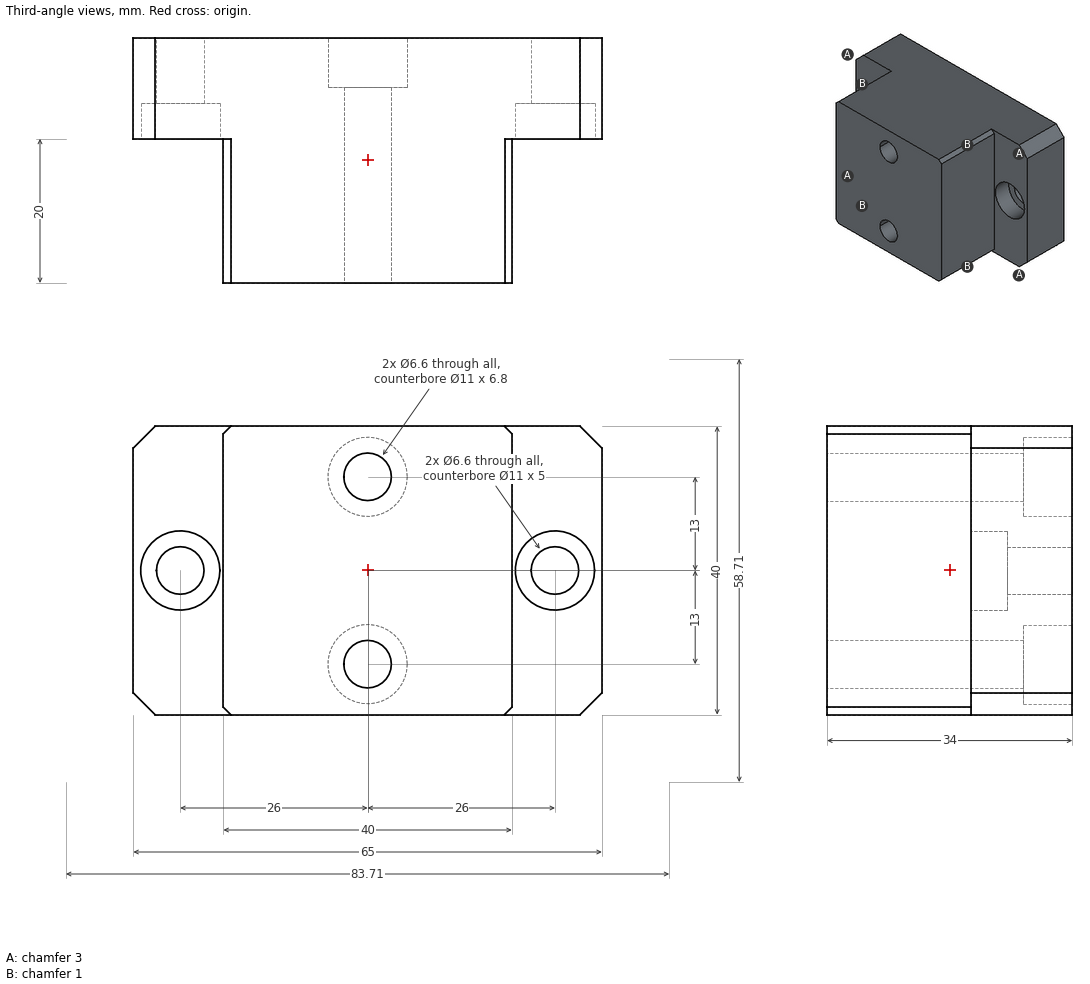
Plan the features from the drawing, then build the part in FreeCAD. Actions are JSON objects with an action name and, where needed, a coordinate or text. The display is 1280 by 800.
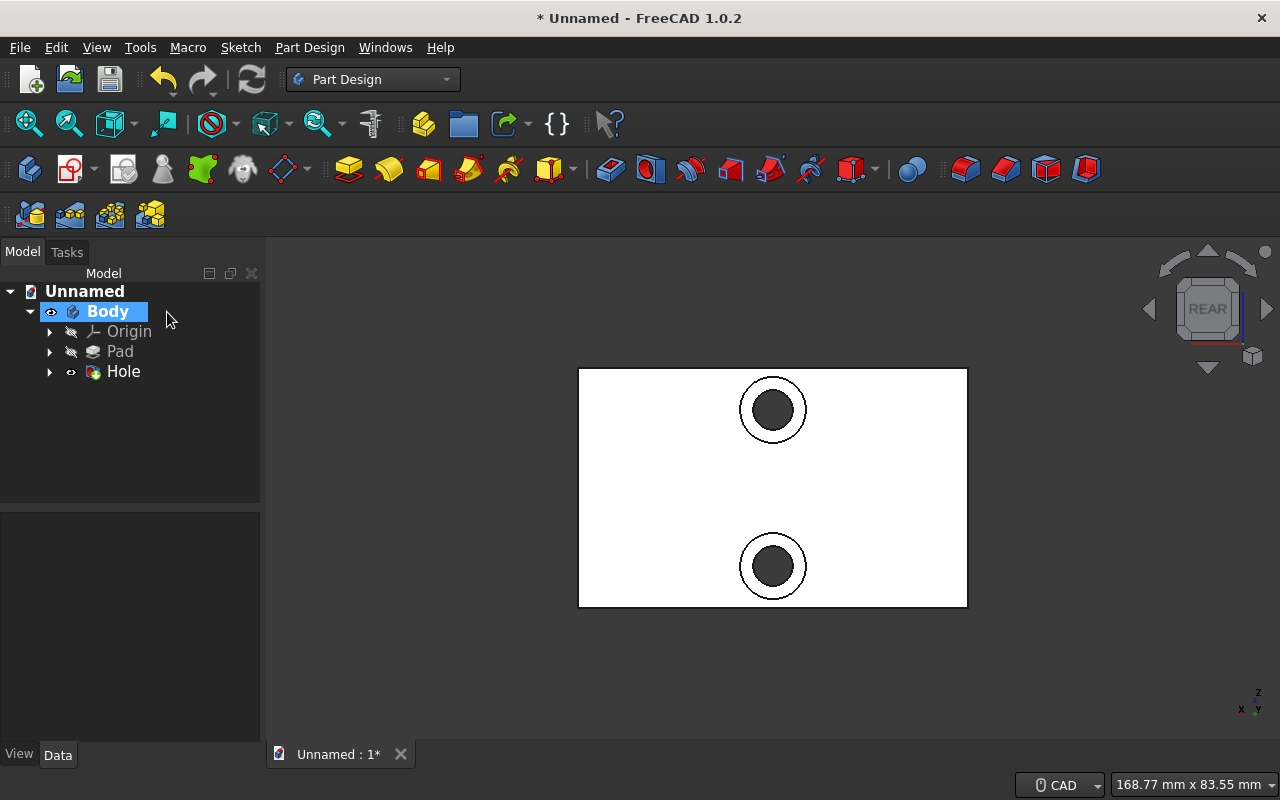
{"action": "key", "text": "0"}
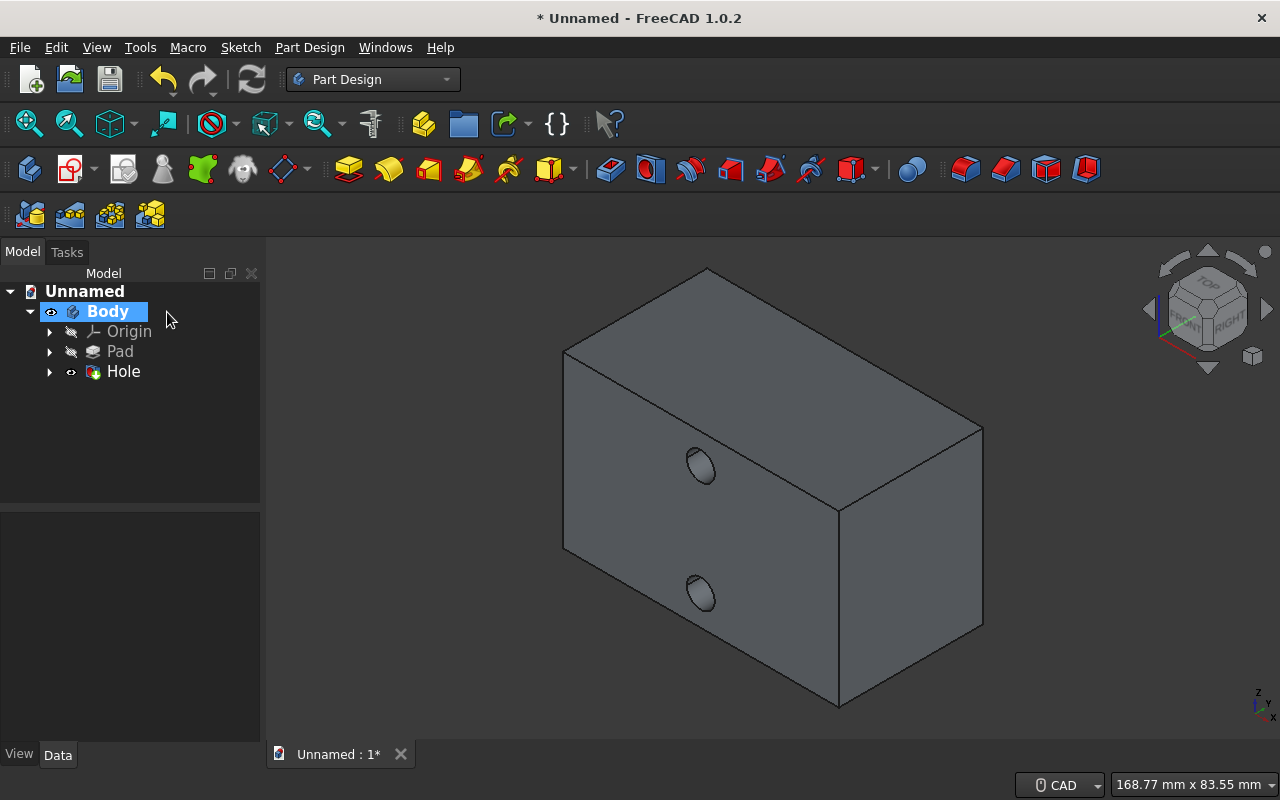
{"action": "left_click", "coordinate": [911, 469]}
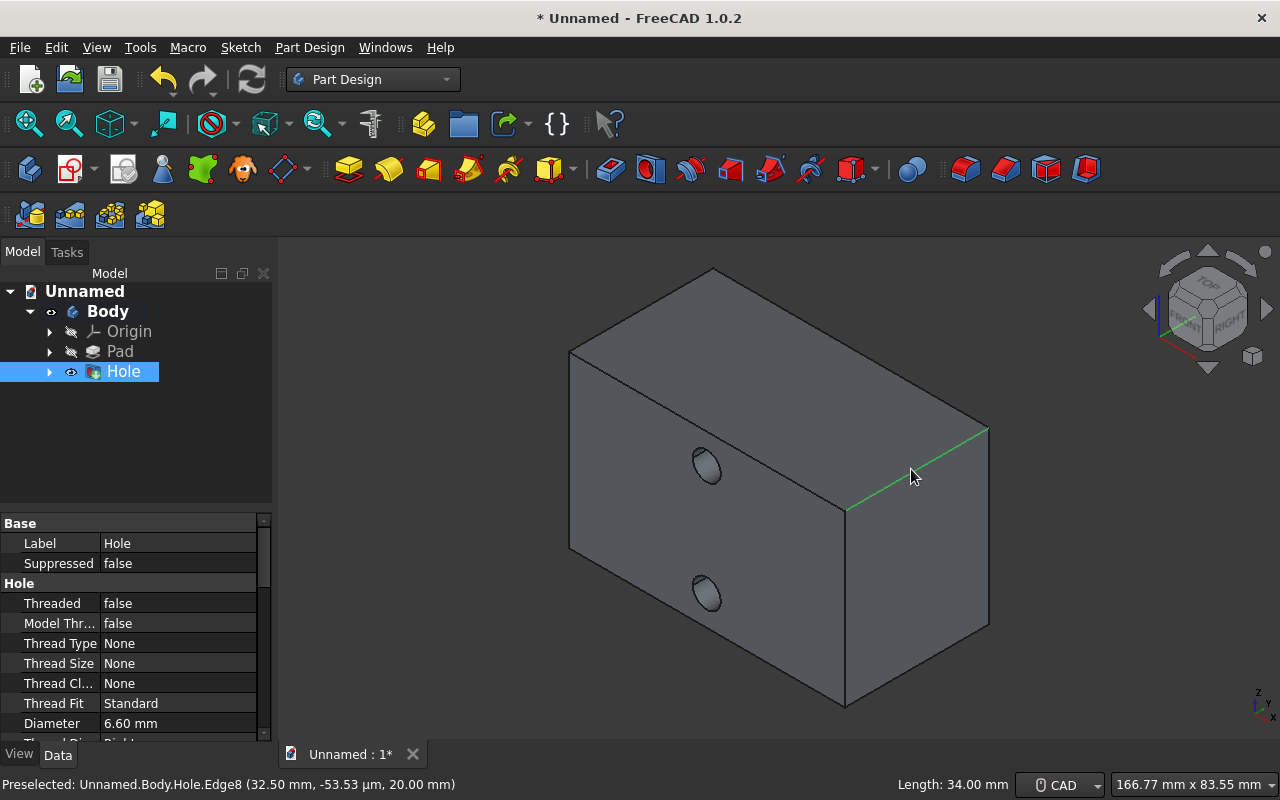
{"action": "key", "text": "2"}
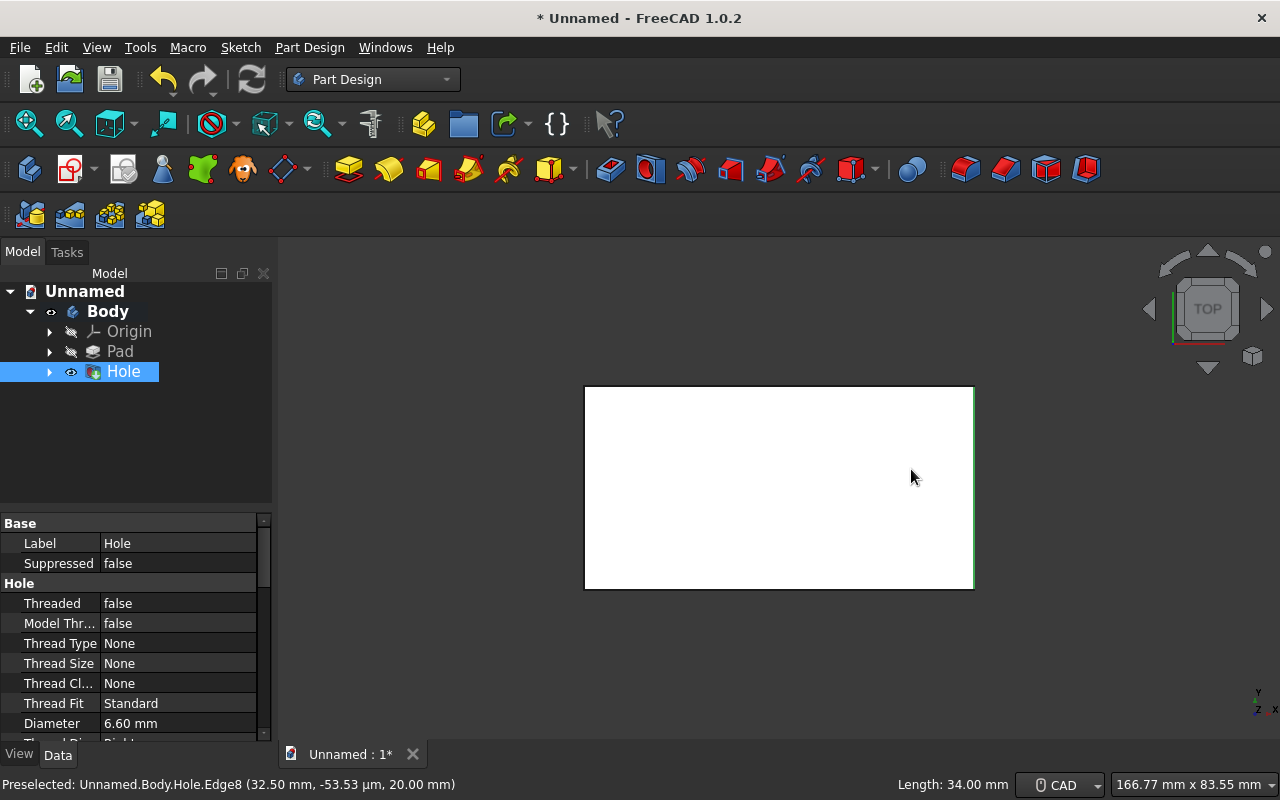
{"action": "left_click", "coordinate": [30, 124]}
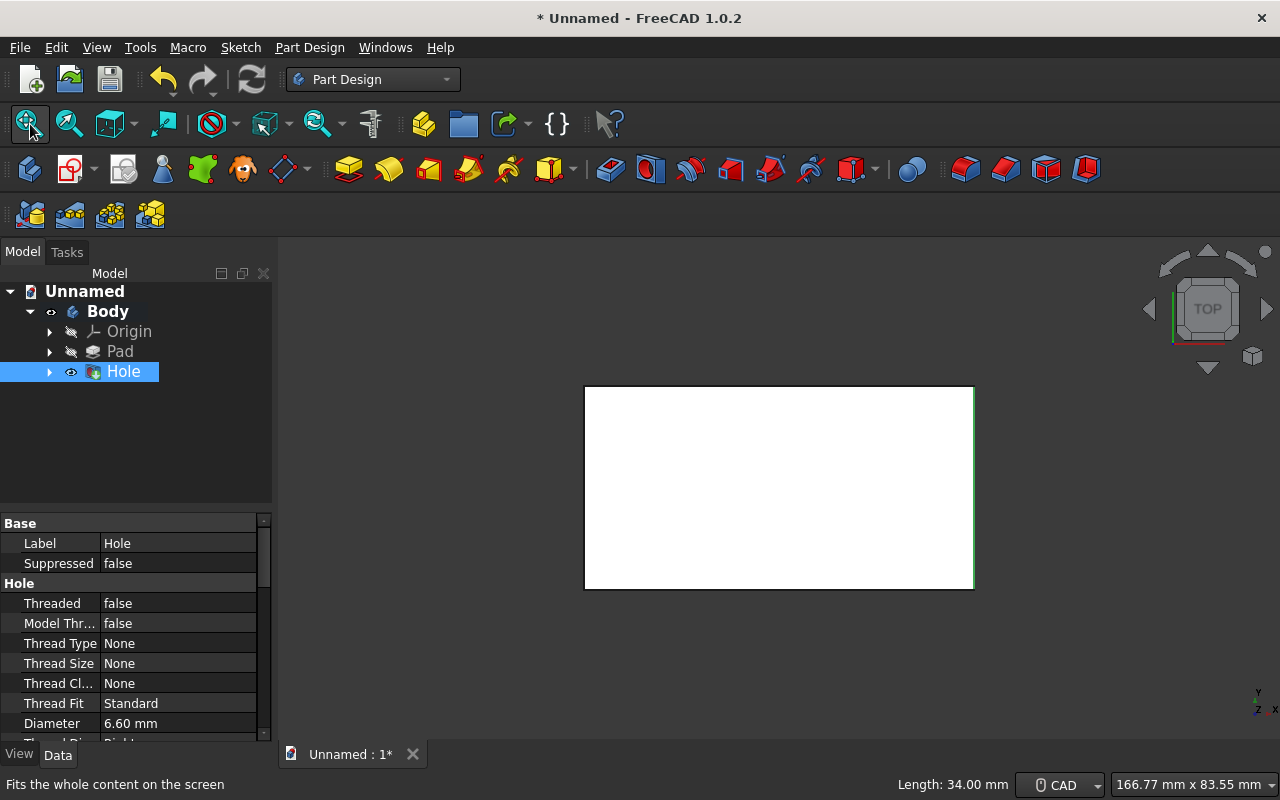
{"action": "left_click", "coordinate": [584, 487], "text": "ctrl"}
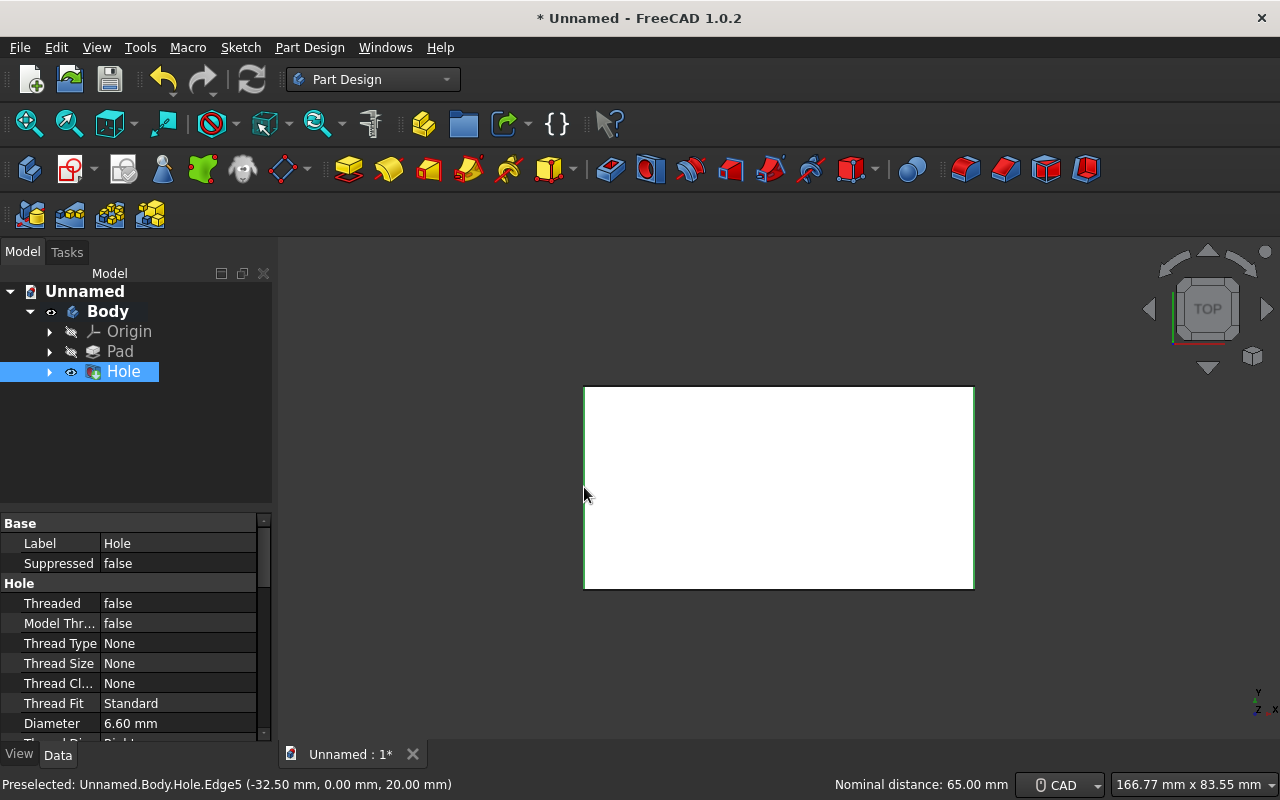
{"action": "key", "text": "1"}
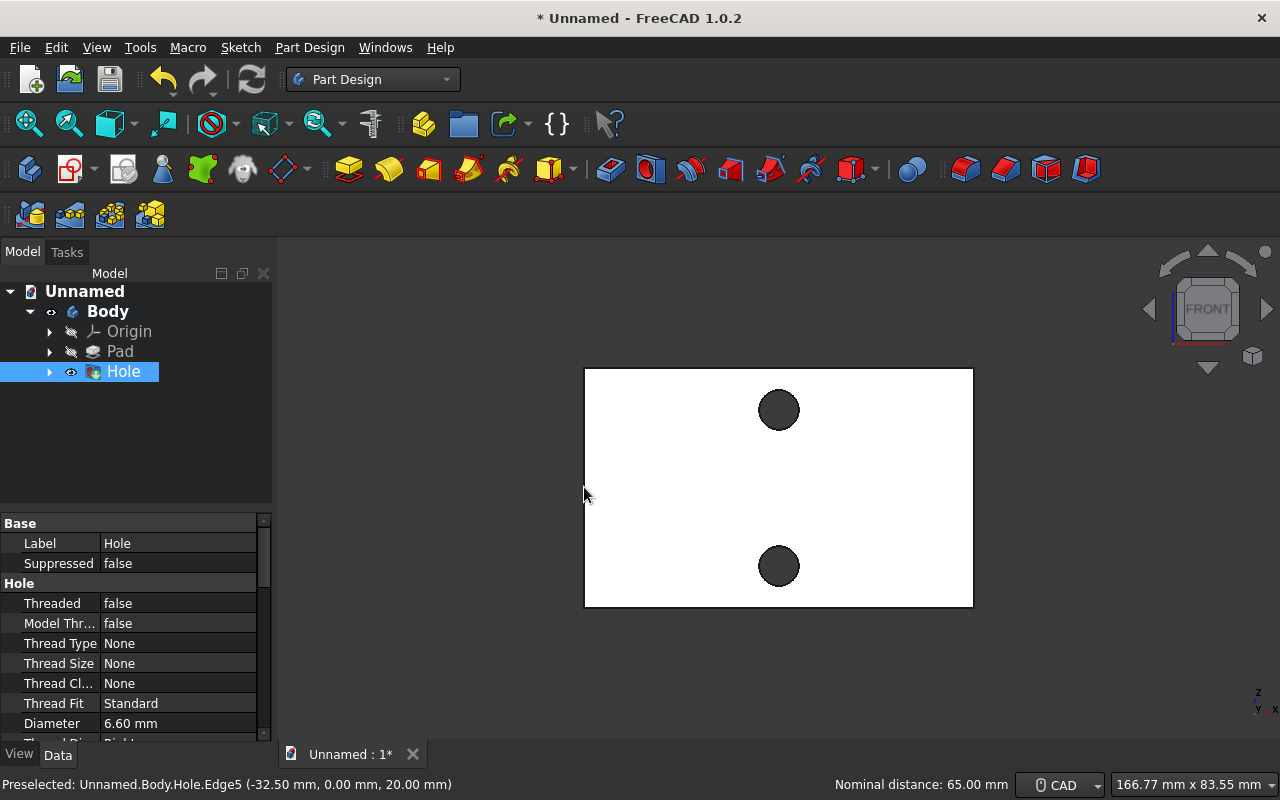
{"action": "key", "text": "3"}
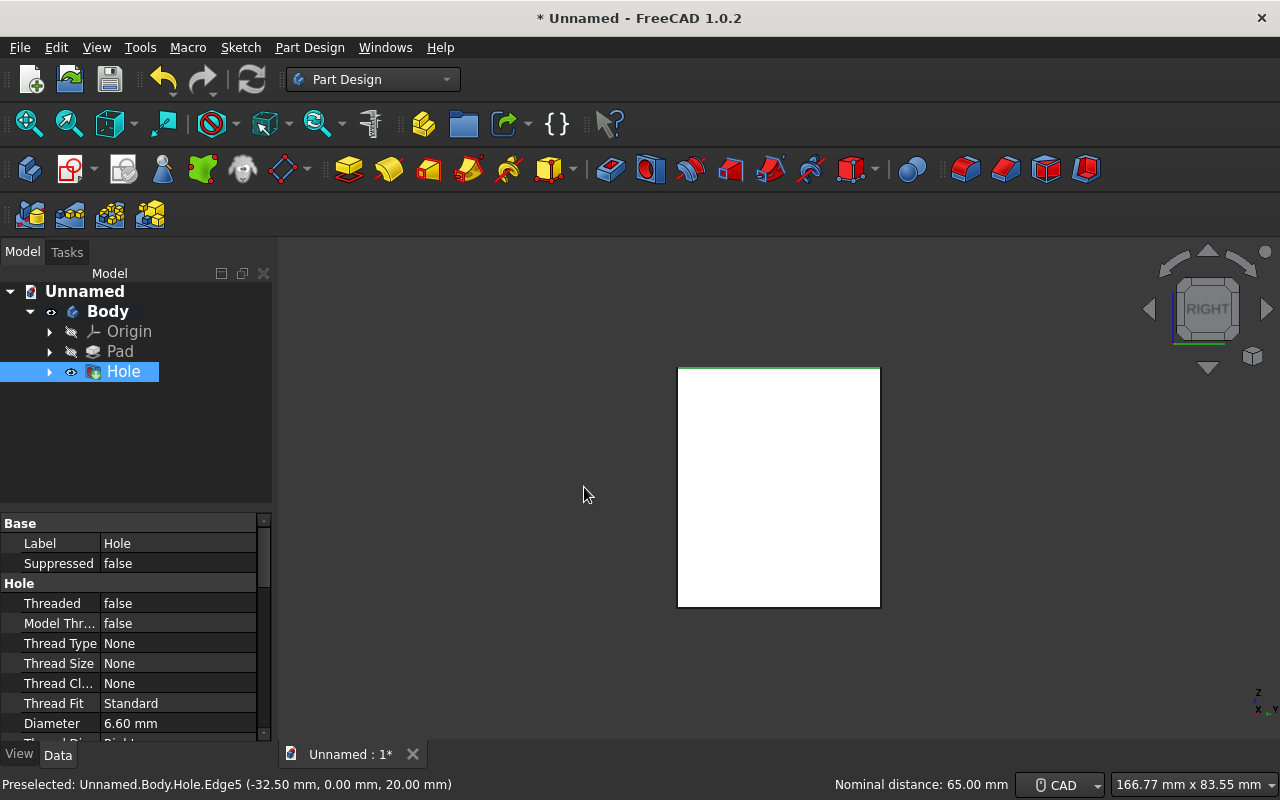
{"action": "left_click", "coordinate": [779, 607], "text": "ctrl"}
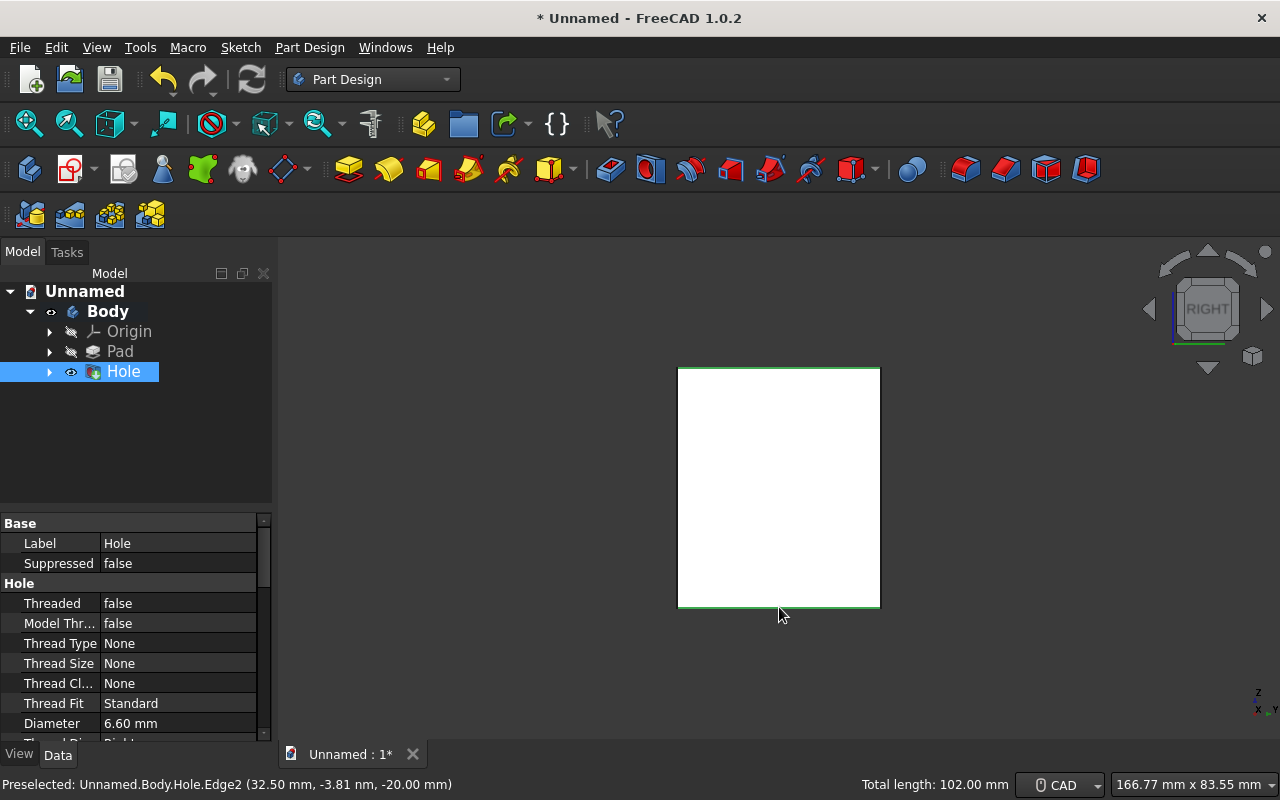
{"action": "key", "text": "5"}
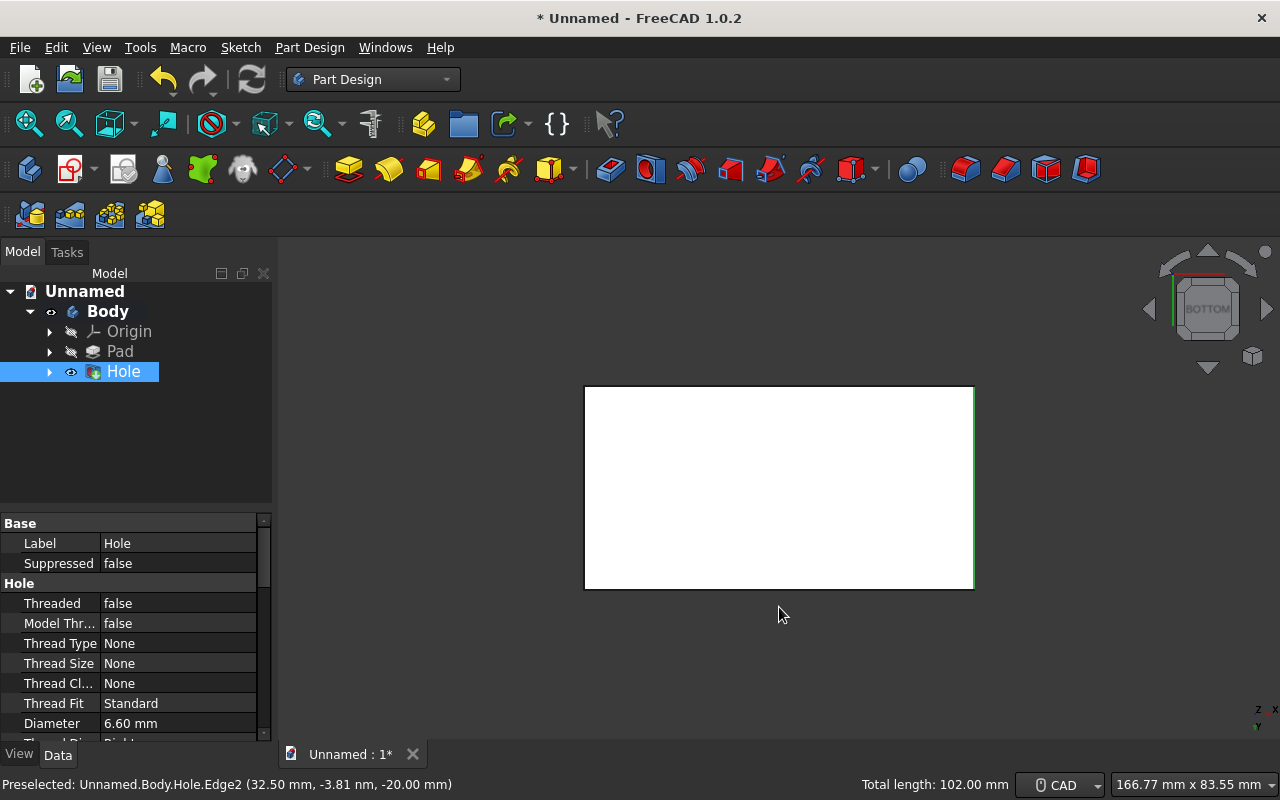
{"action": "left_click", "coordinate": [30, 124]}